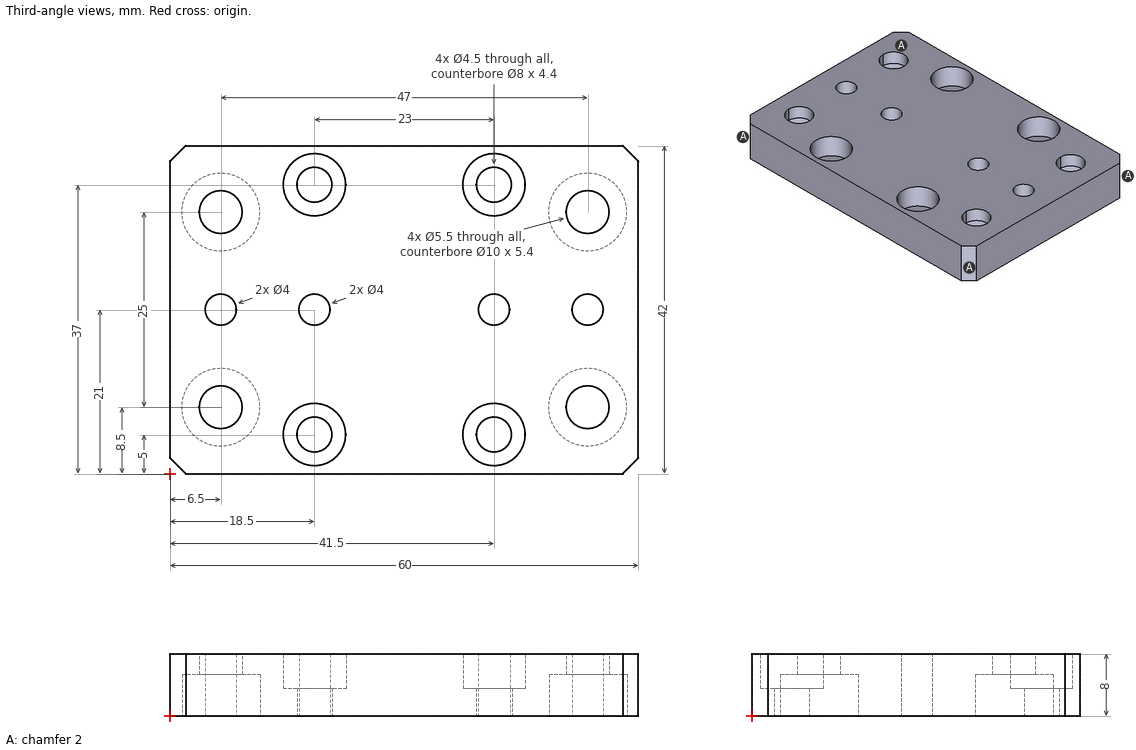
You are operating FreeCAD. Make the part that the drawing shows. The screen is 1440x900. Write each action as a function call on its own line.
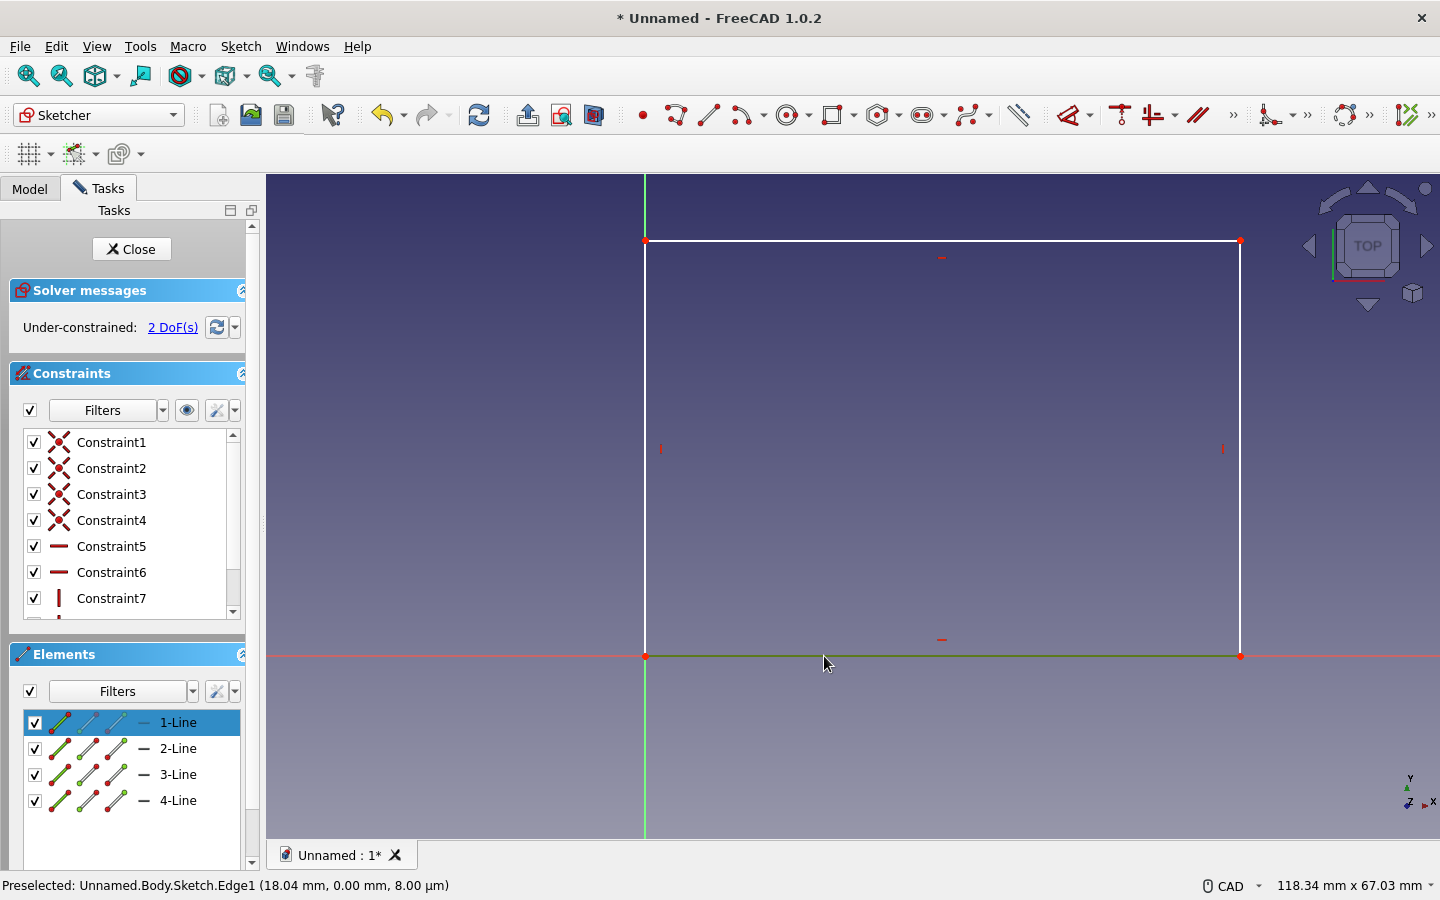
key(l)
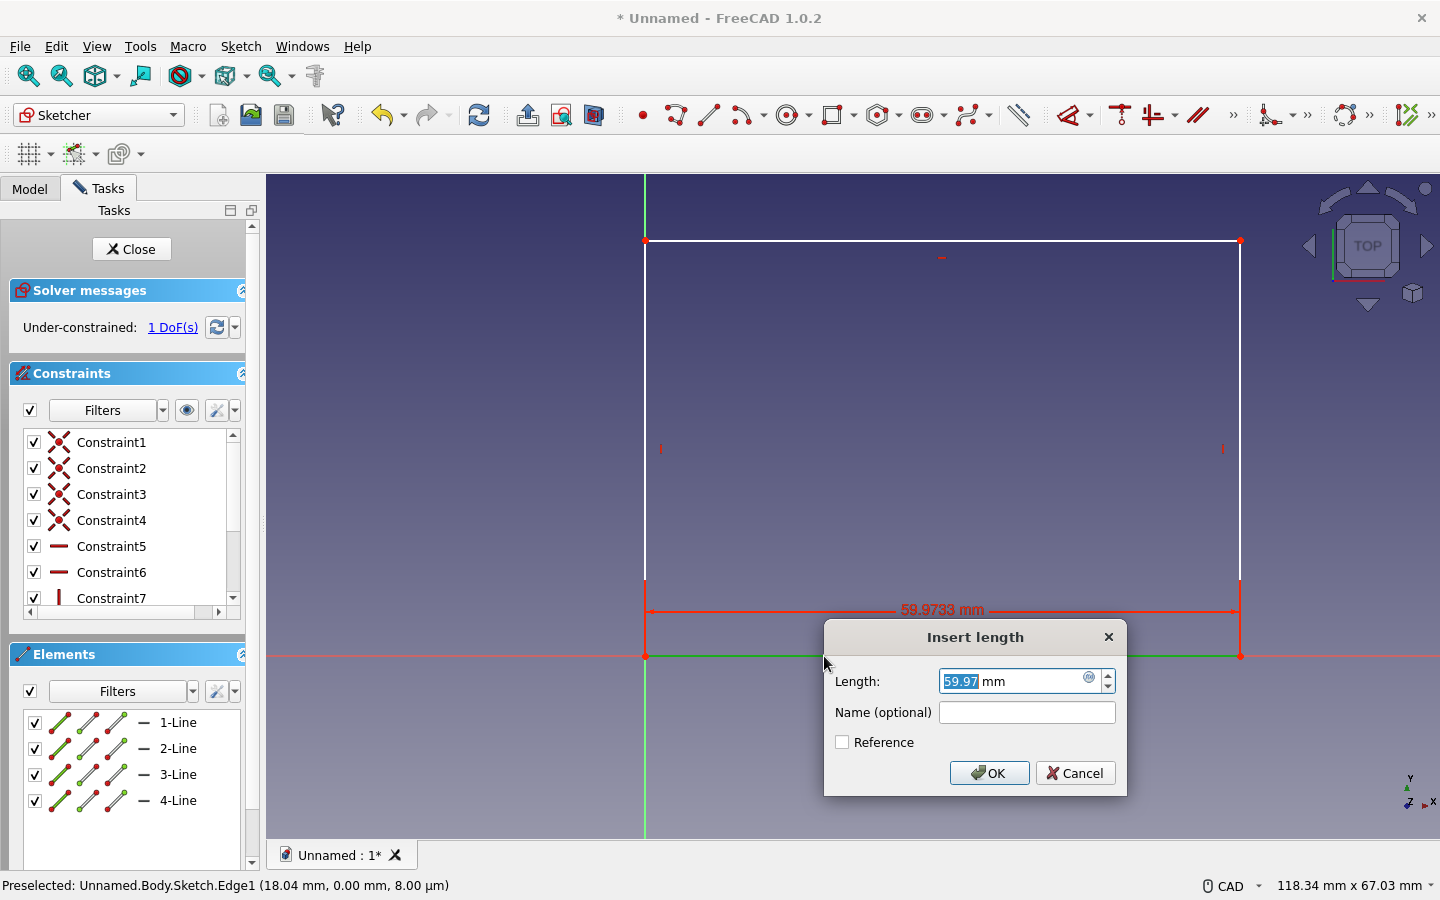
text(60)
key(Return)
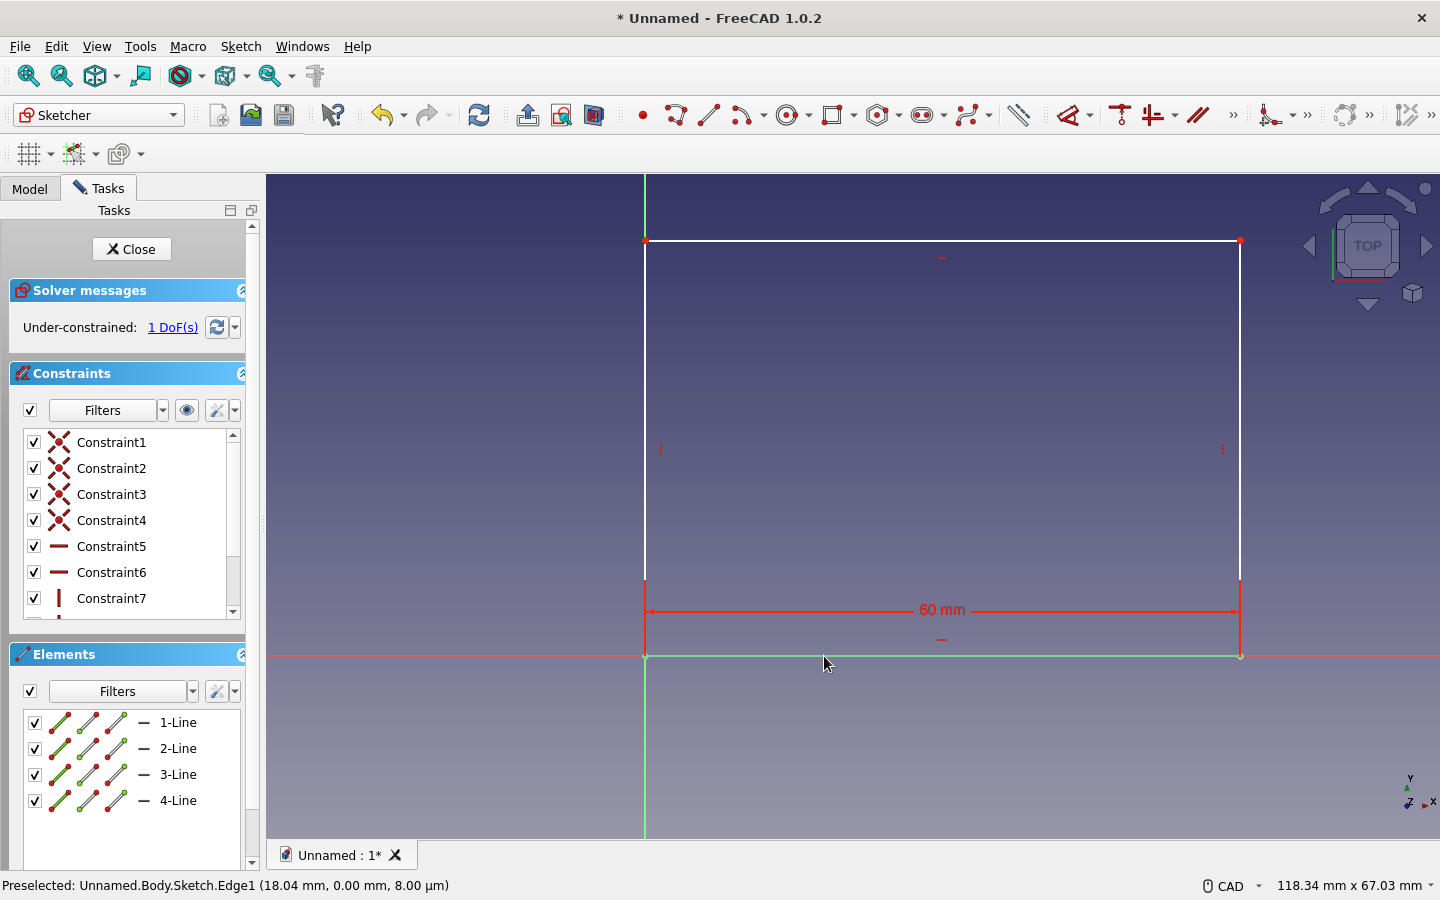
click(1240, 532)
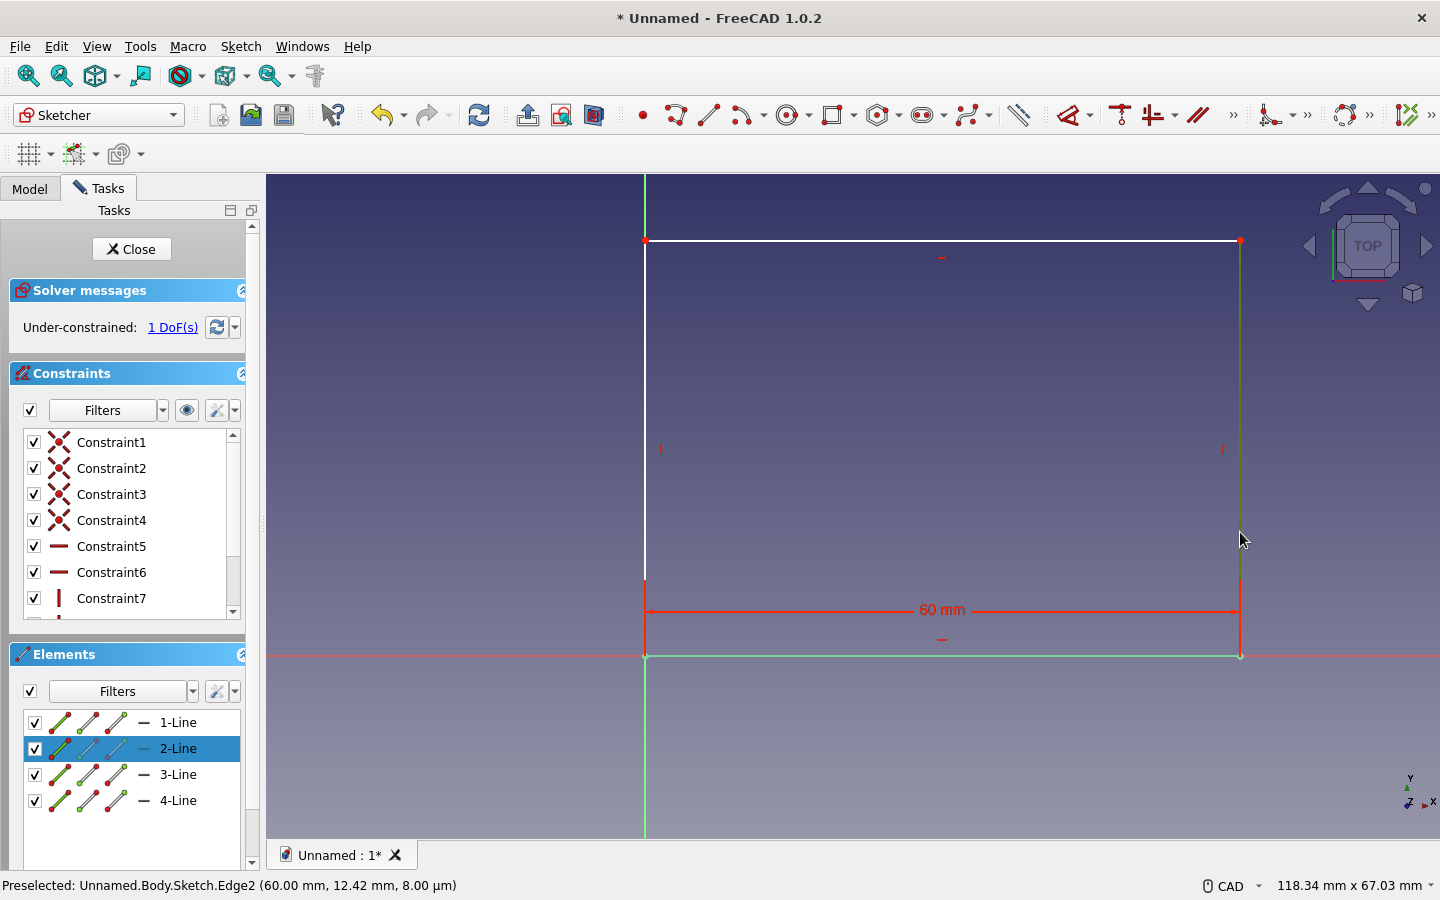
key(i)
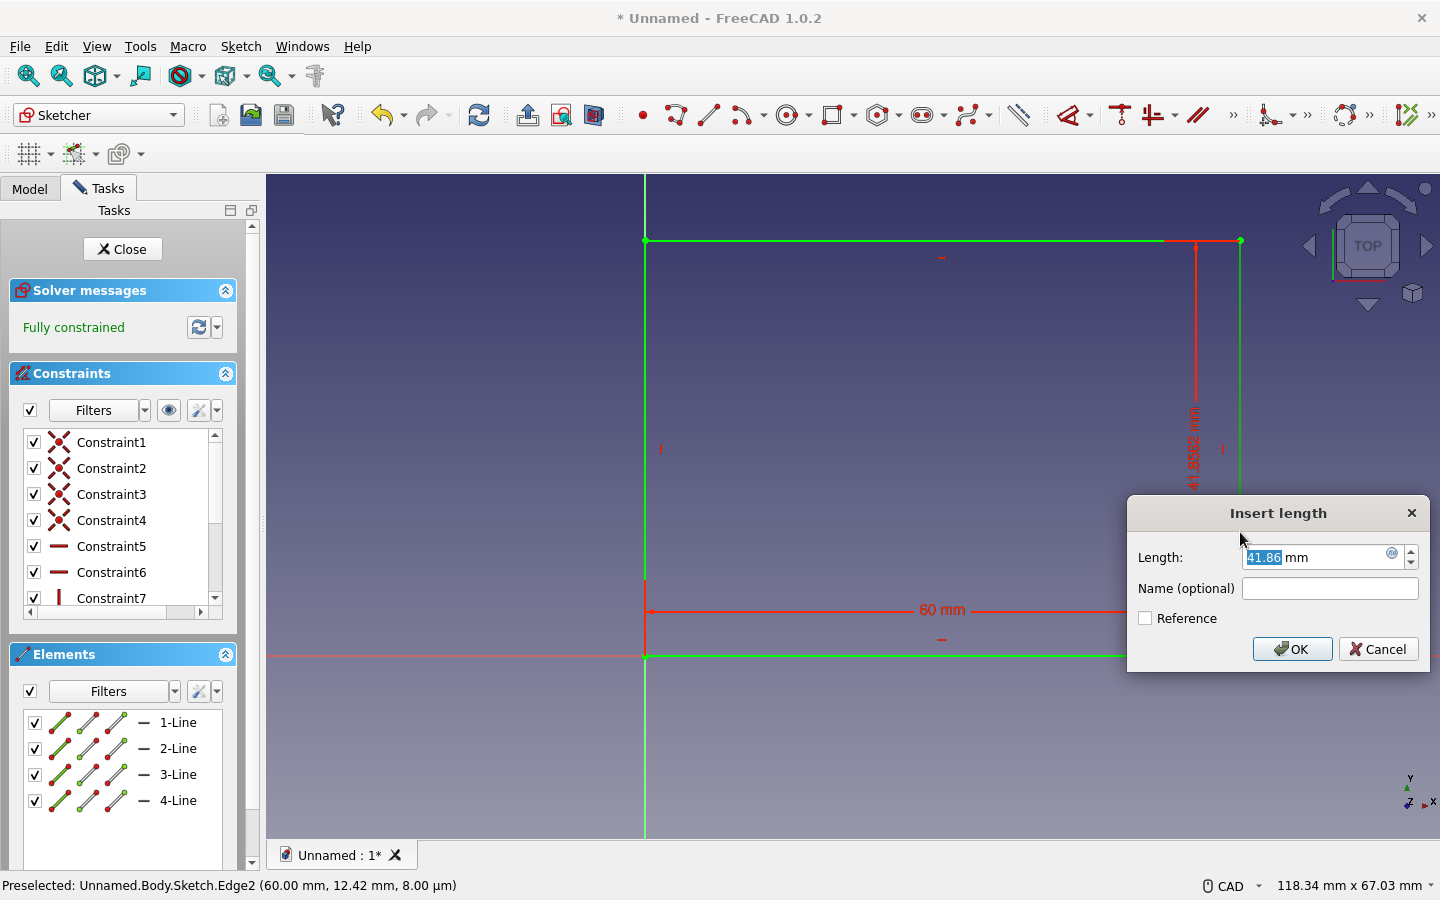
text(42)
key(Return)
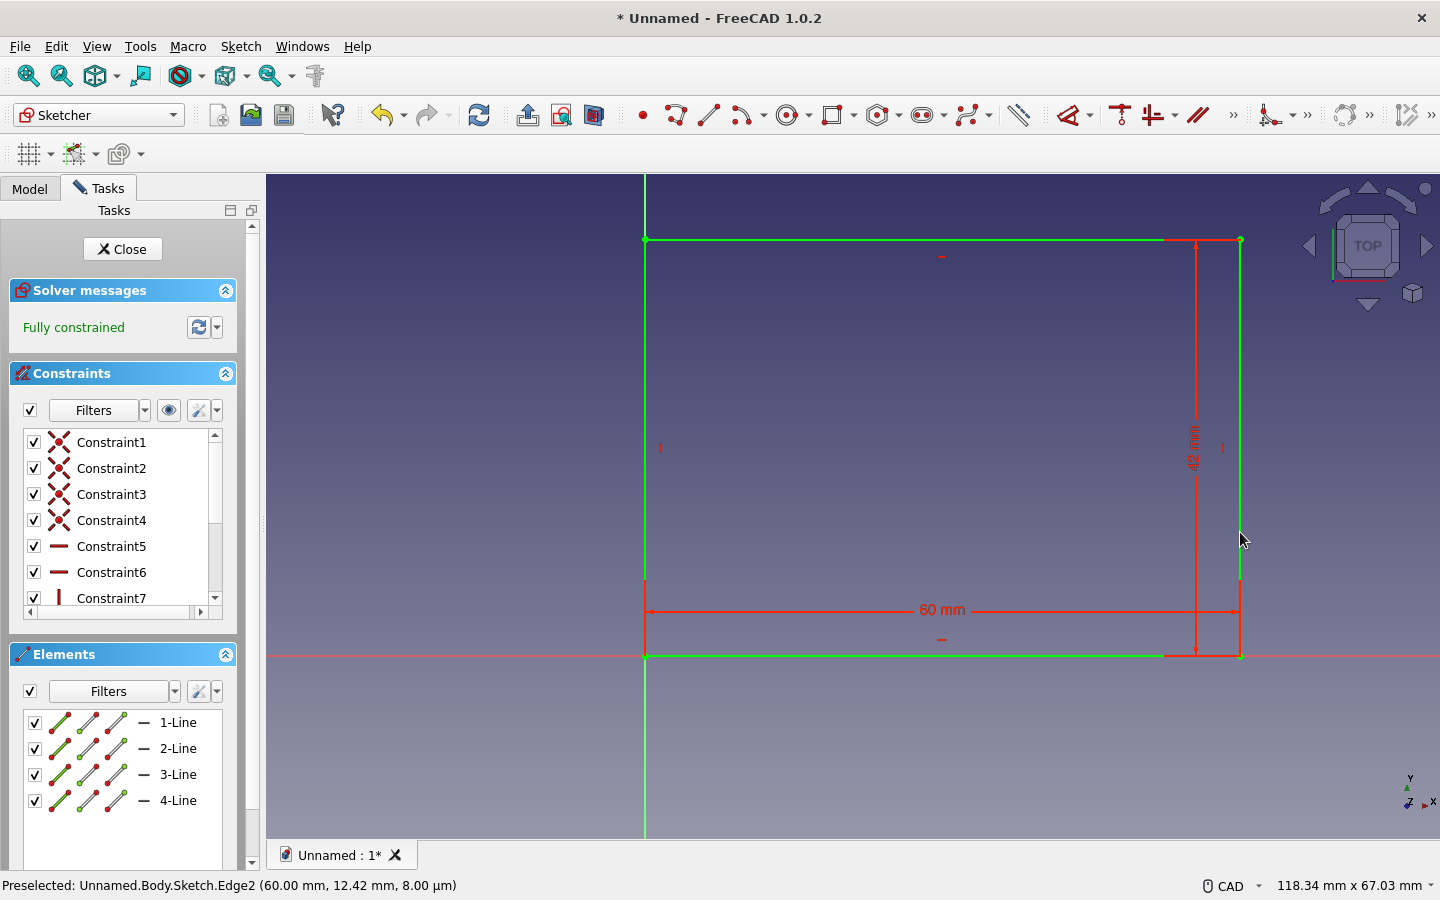
click(123, 249)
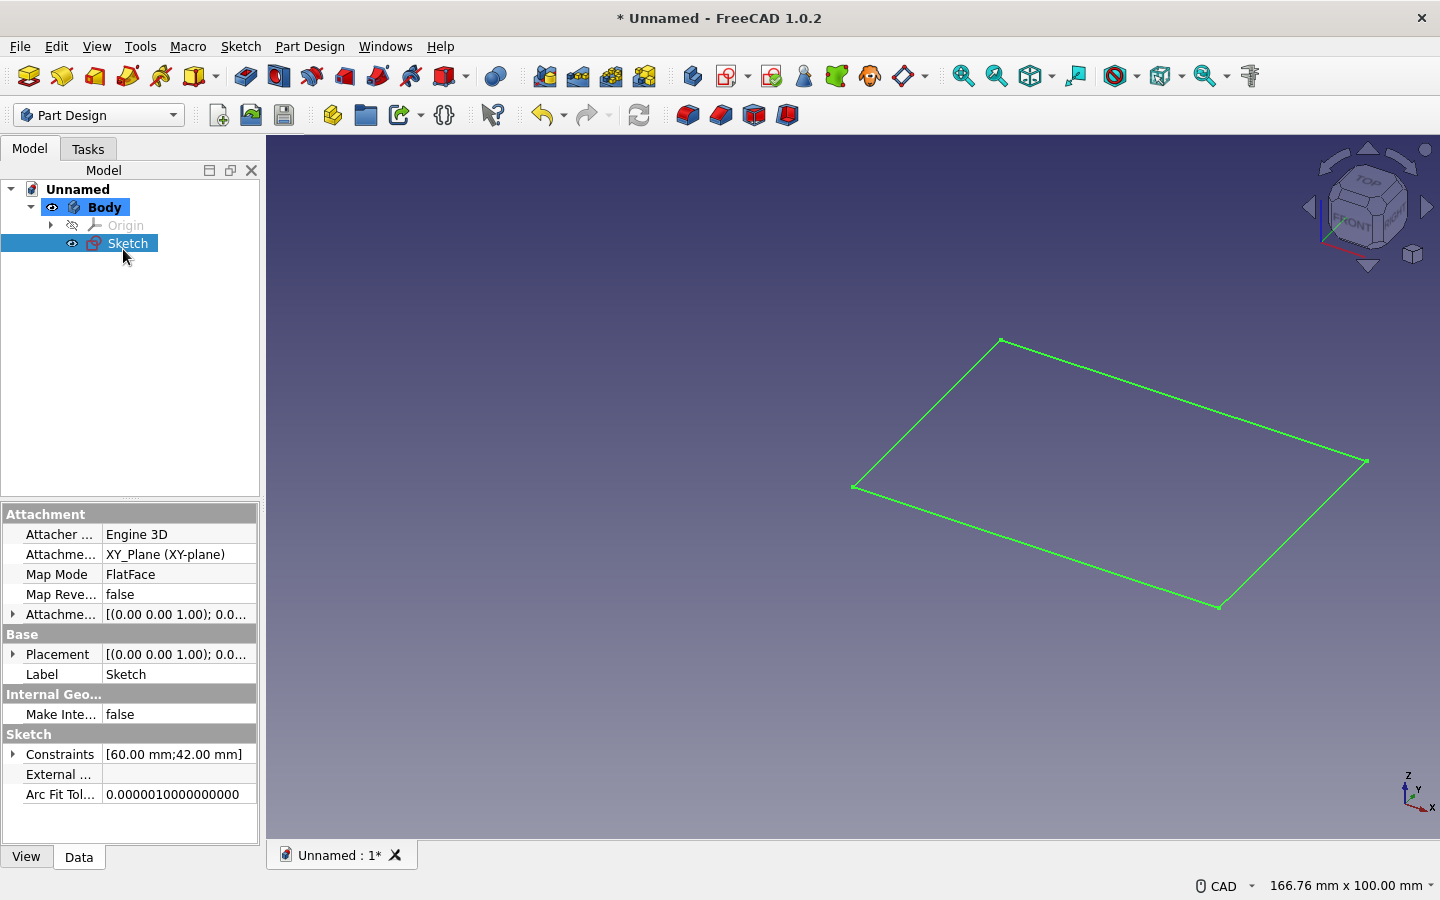
click(29, 76)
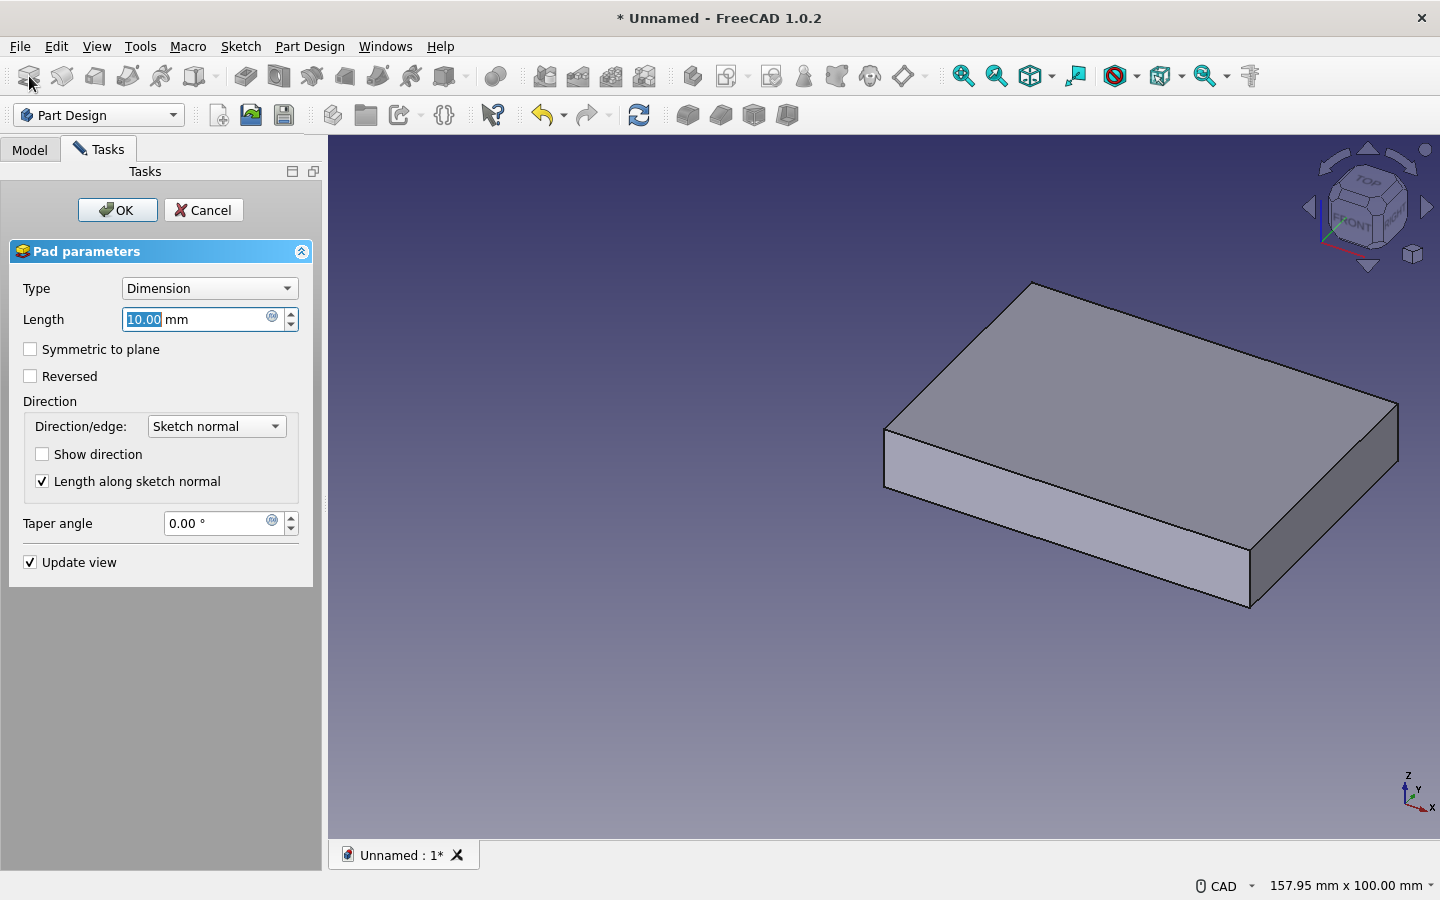
text(8)
key(Tab)